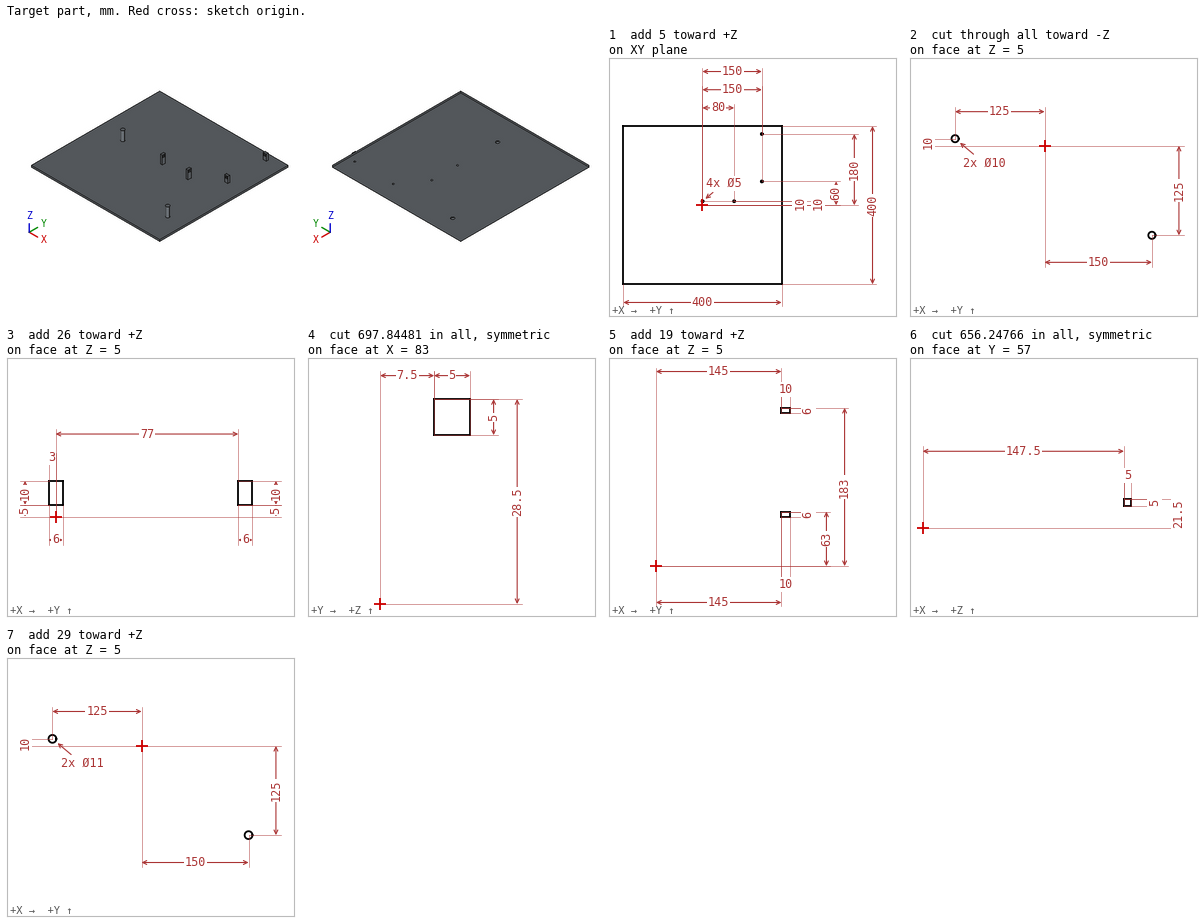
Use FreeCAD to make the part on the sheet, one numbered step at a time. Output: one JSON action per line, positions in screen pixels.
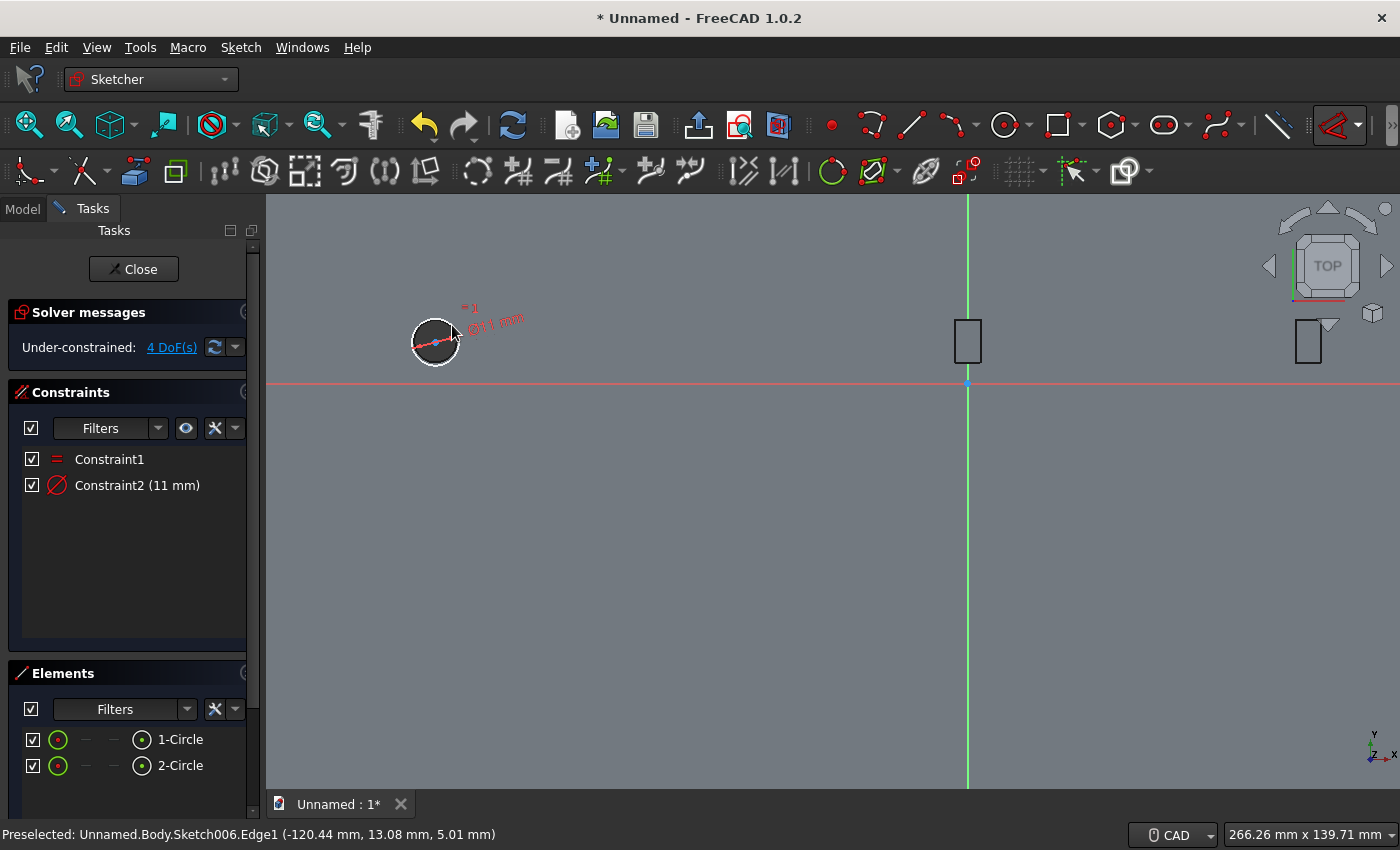
{"action": "left_click", "coordinate": [435, 342]}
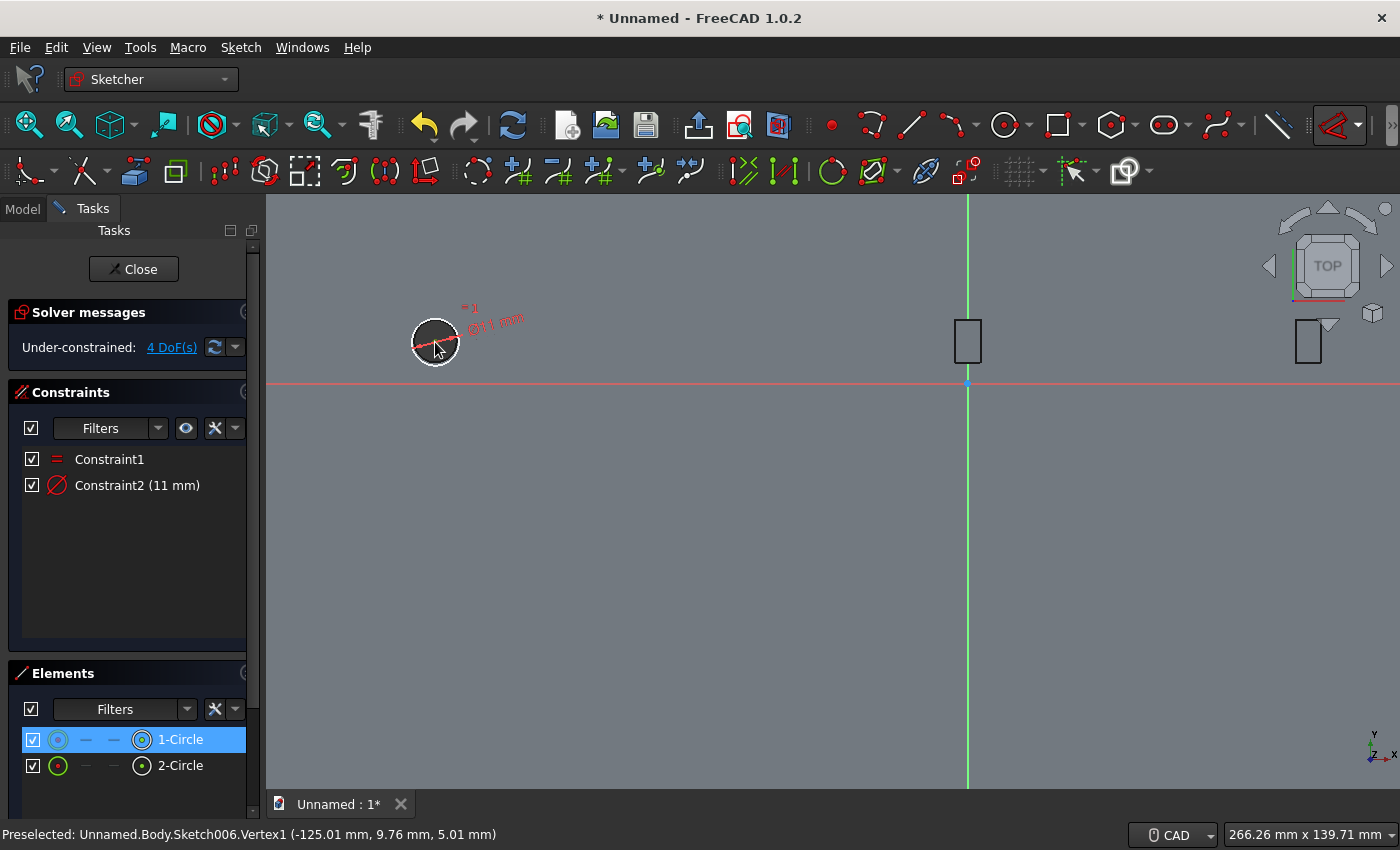
{"action": "key", "text": "i"}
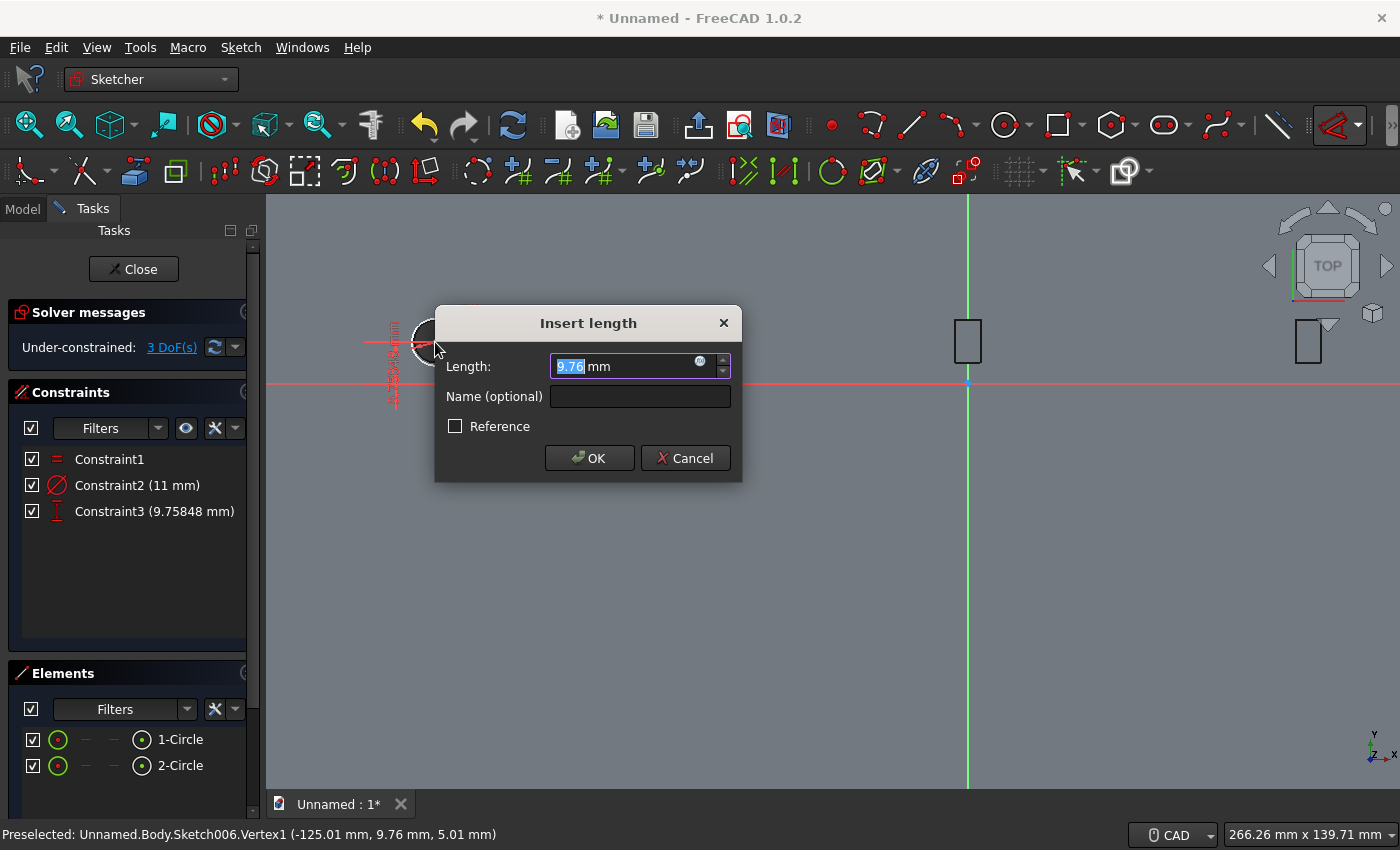
{"action": "type", "text": "10"}
{"action": "key", "text": "Return"}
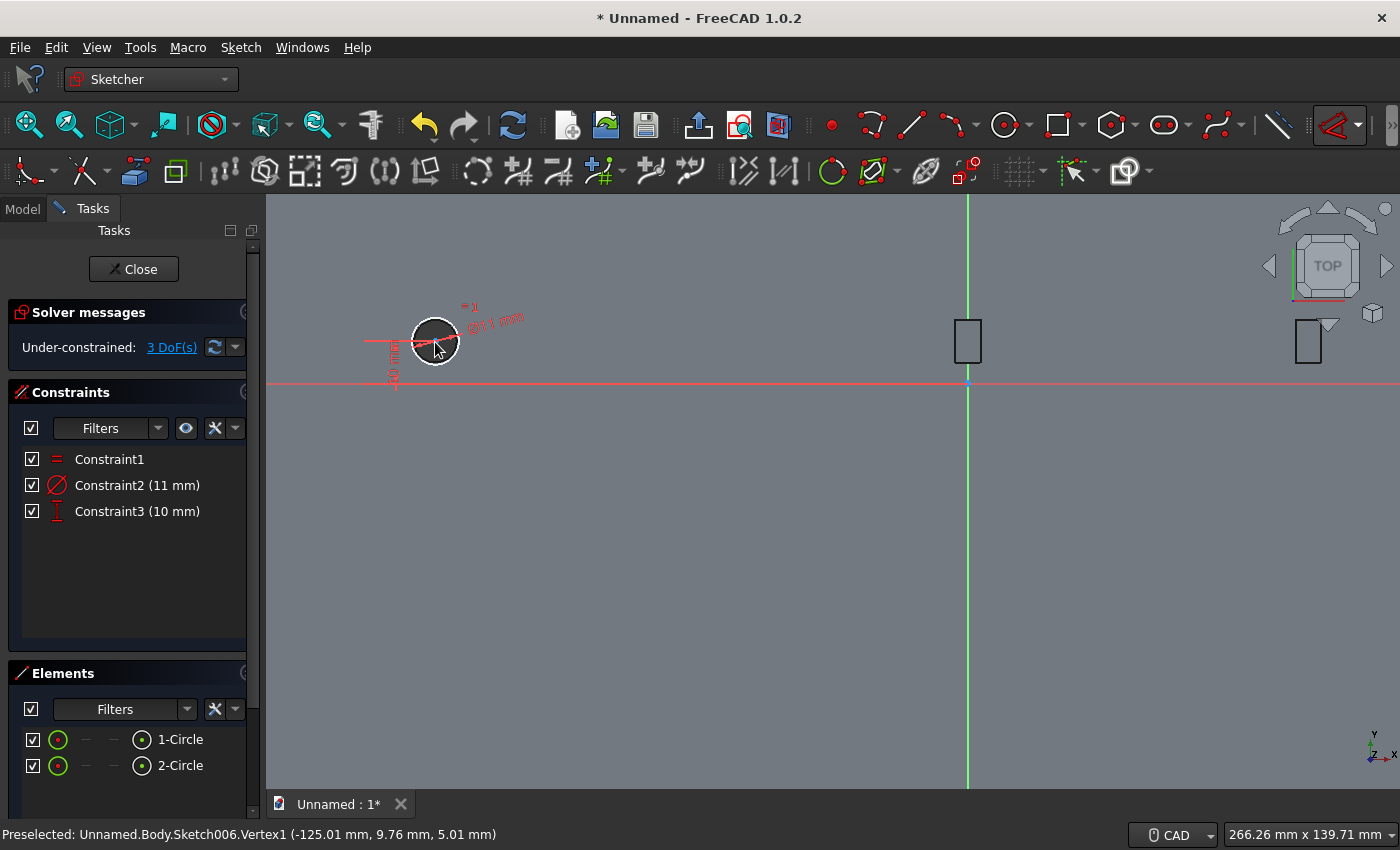
{"action": "left_click", "coordinate": [435, 341]}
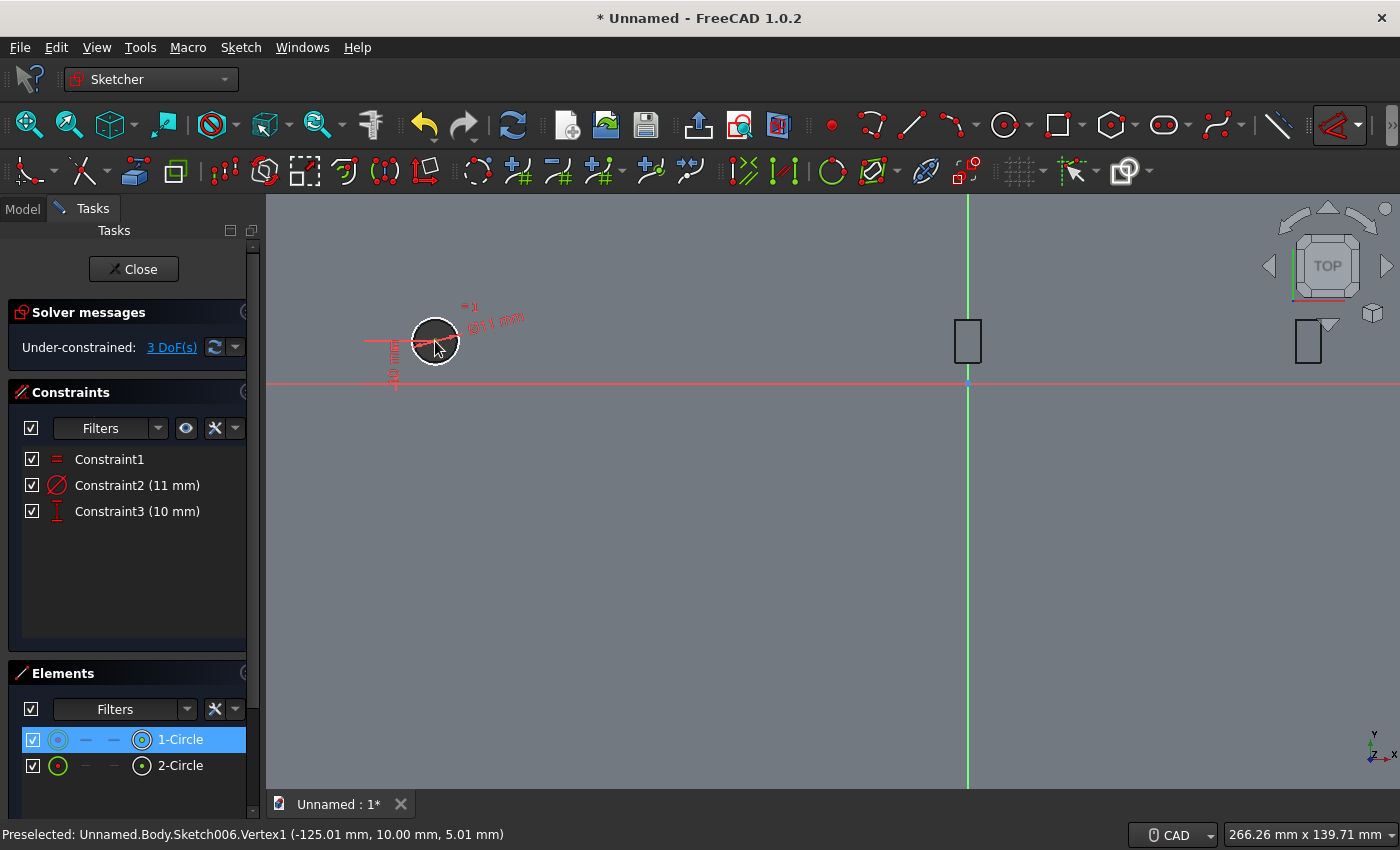
{"action": "key", "text": "l"}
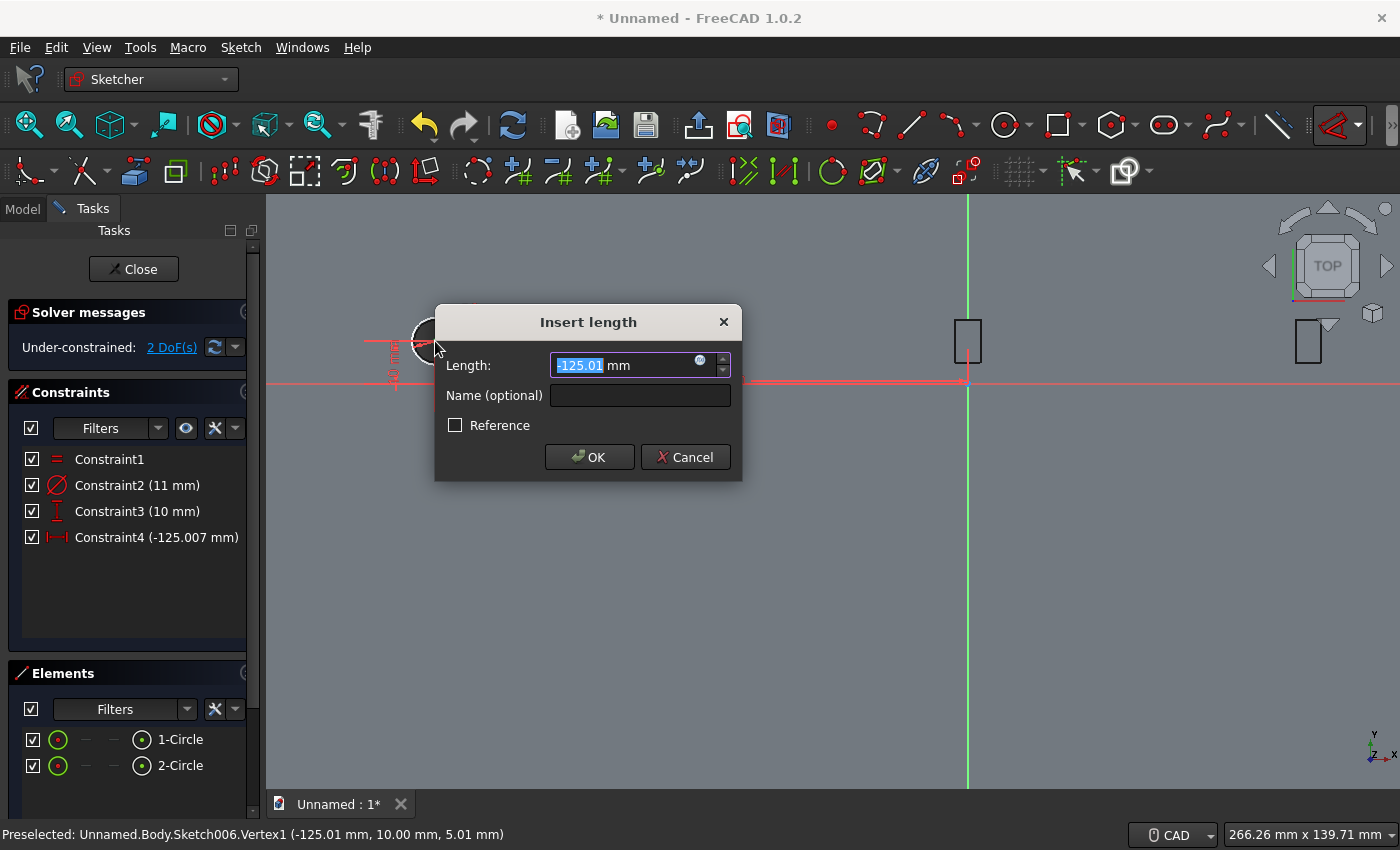
{"action": "type", "text": "-125"}
{"action": "key", "text": "Return"}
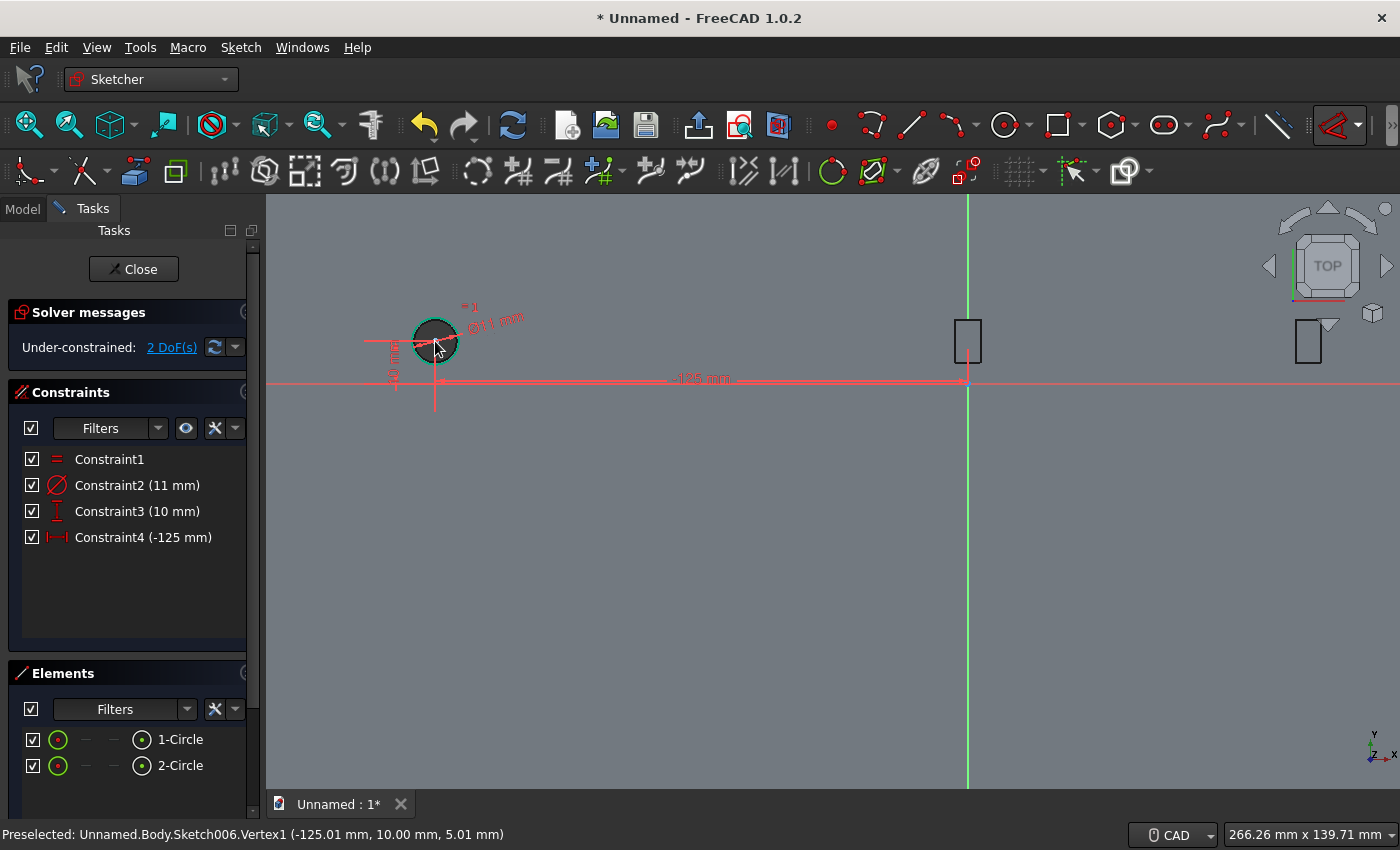
{"action": "scroll", "coordinate": [452, 325], "scroll_direction": "down", "scroll_amount": 3}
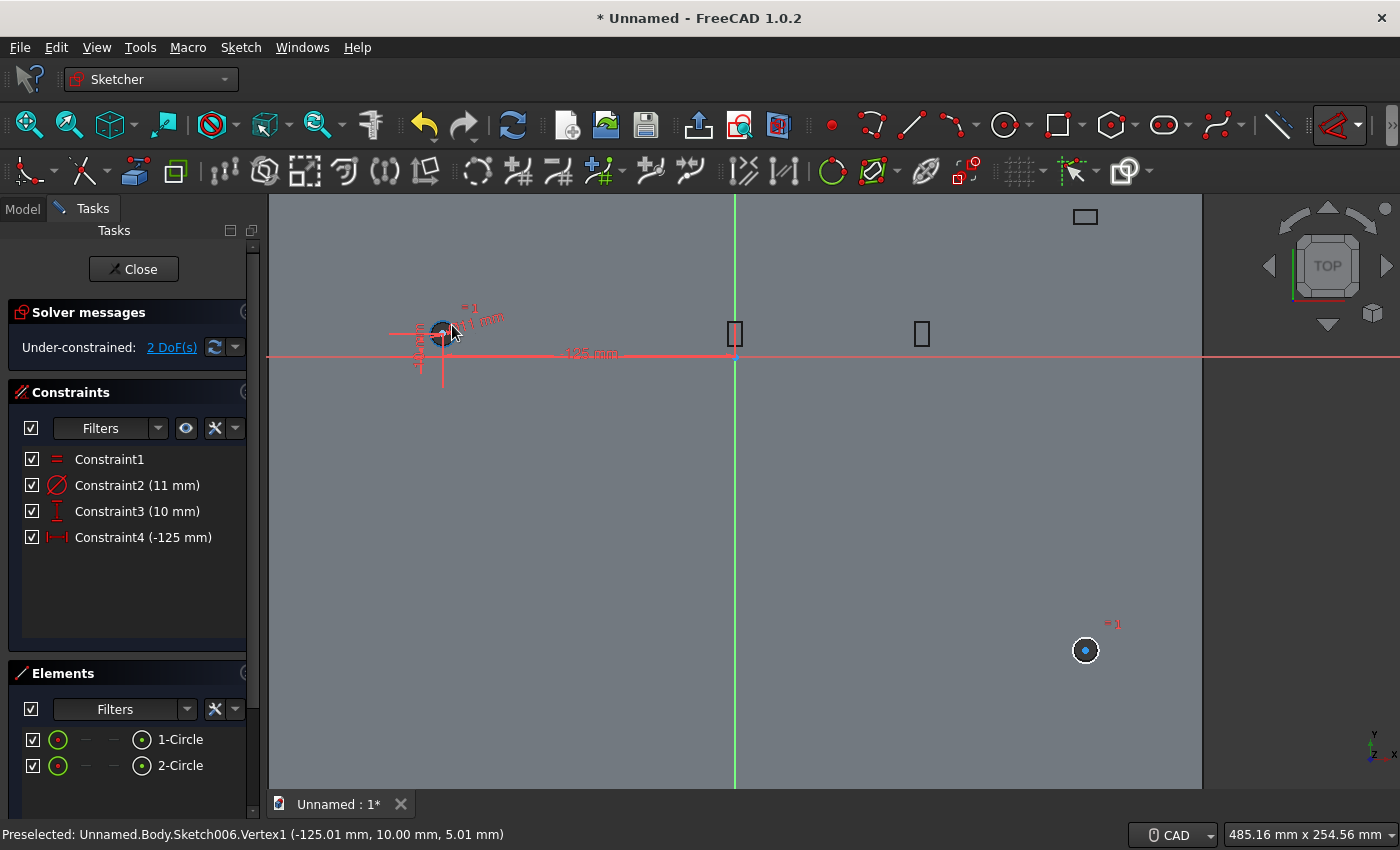
{"action": "left_click", "coordinate": [1086, 650]}